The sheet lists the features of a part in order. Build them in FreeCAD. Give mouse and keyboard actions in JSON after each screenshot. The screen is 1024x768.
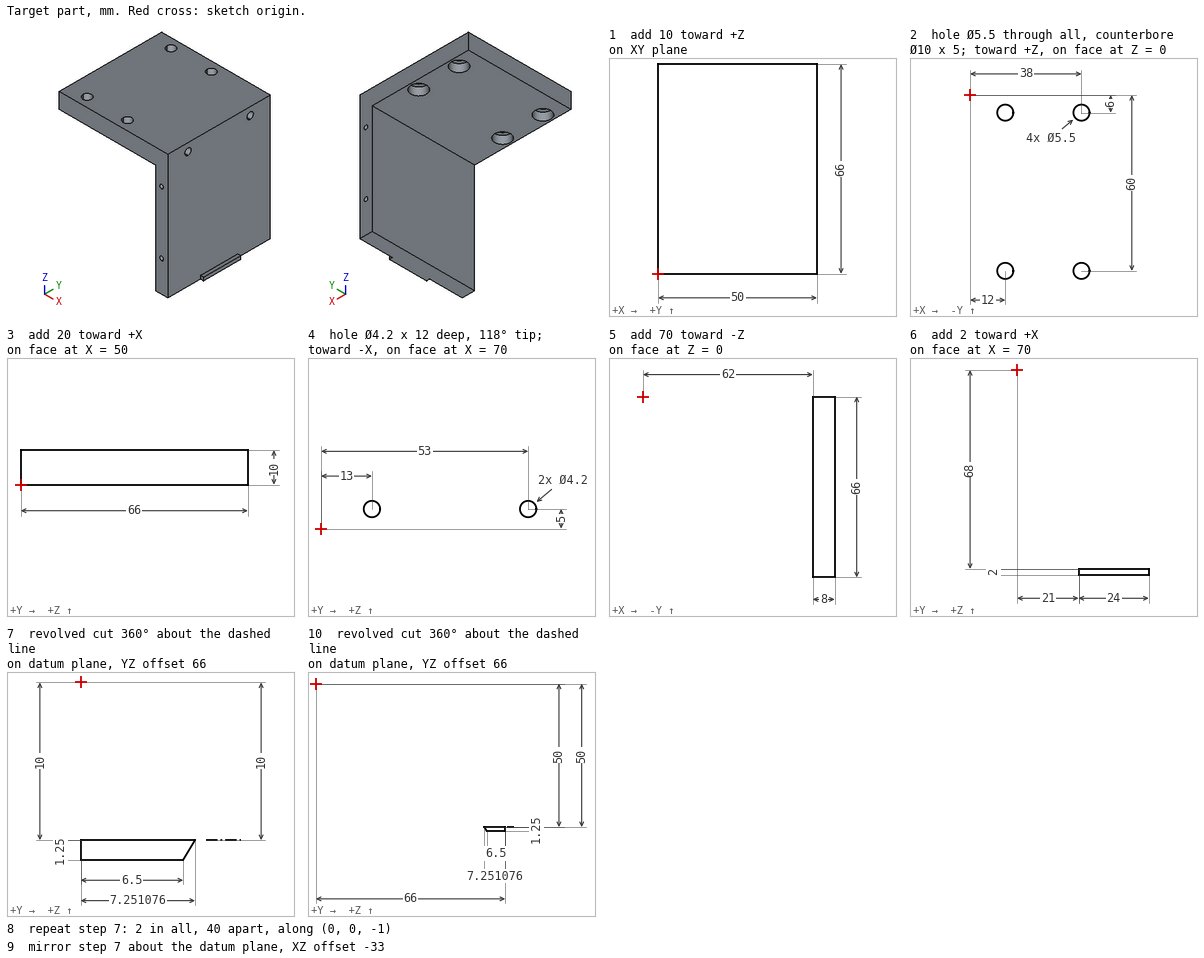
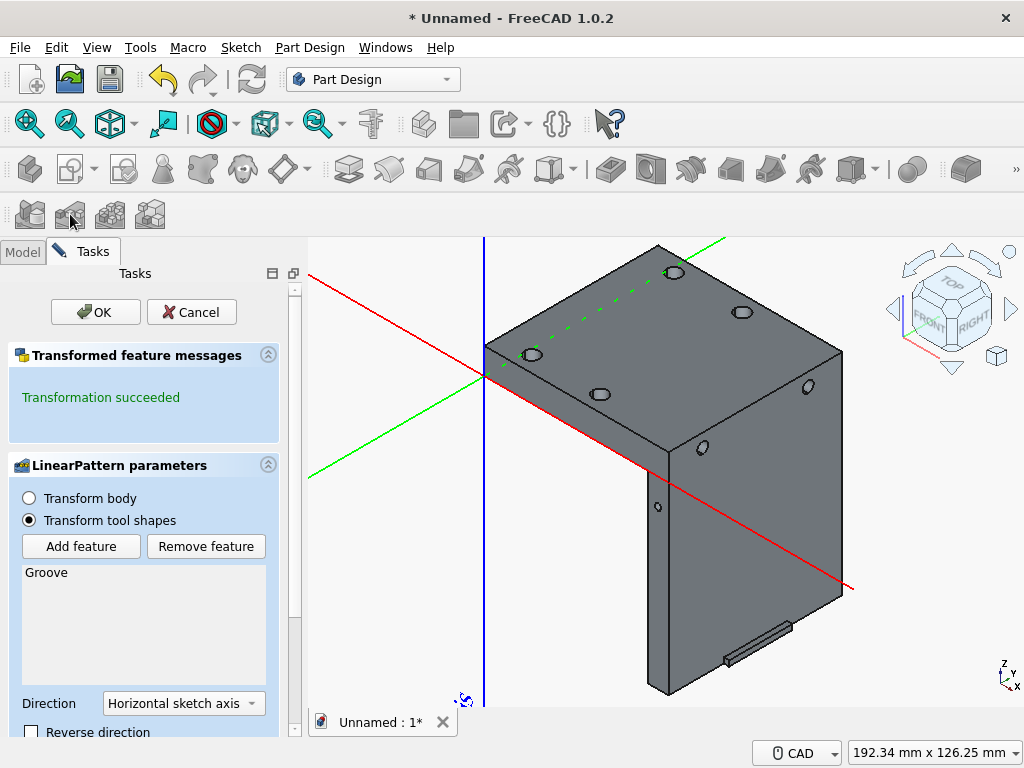
{"action": "left_click", "coordinate": [184, 704]}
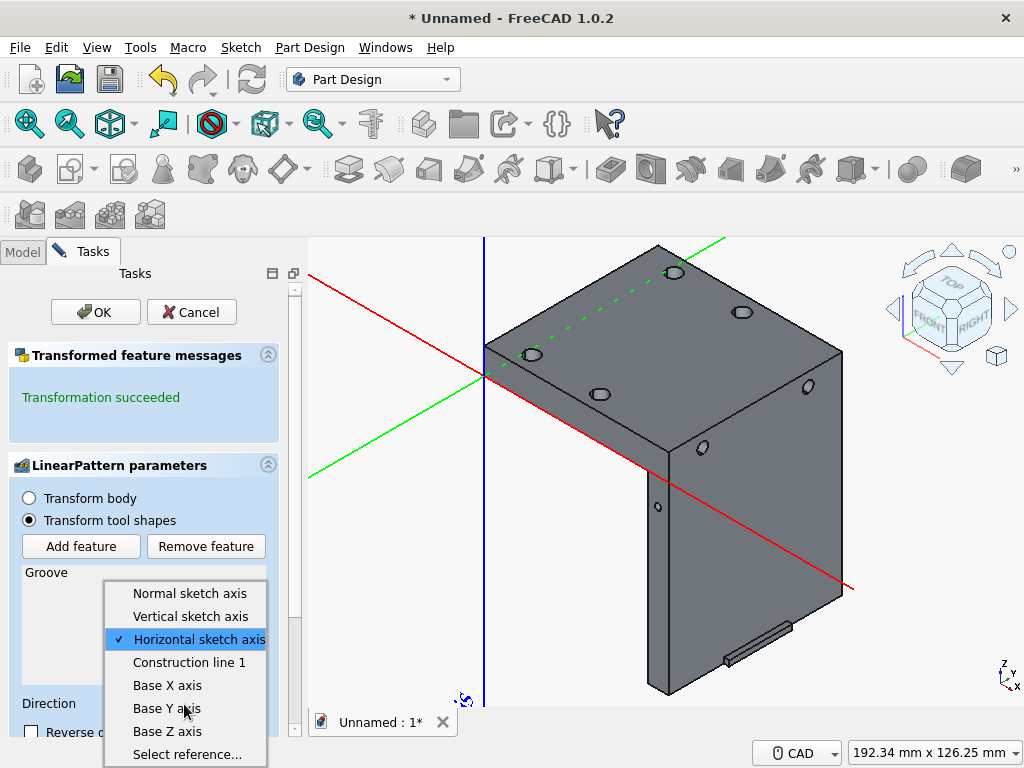
{"action": "left_click", "coordinate": [184, 732]}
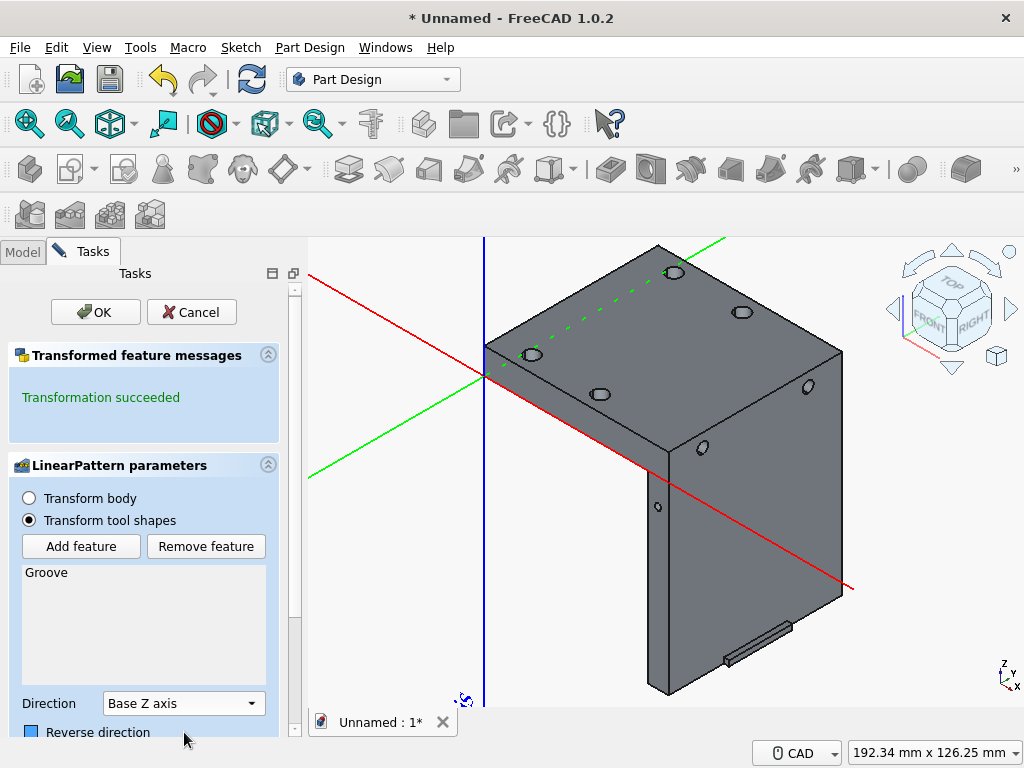
{"action": "scroll", "coordinate": [295, 510], "scroll_direction": "down", "scroll_amount": 2}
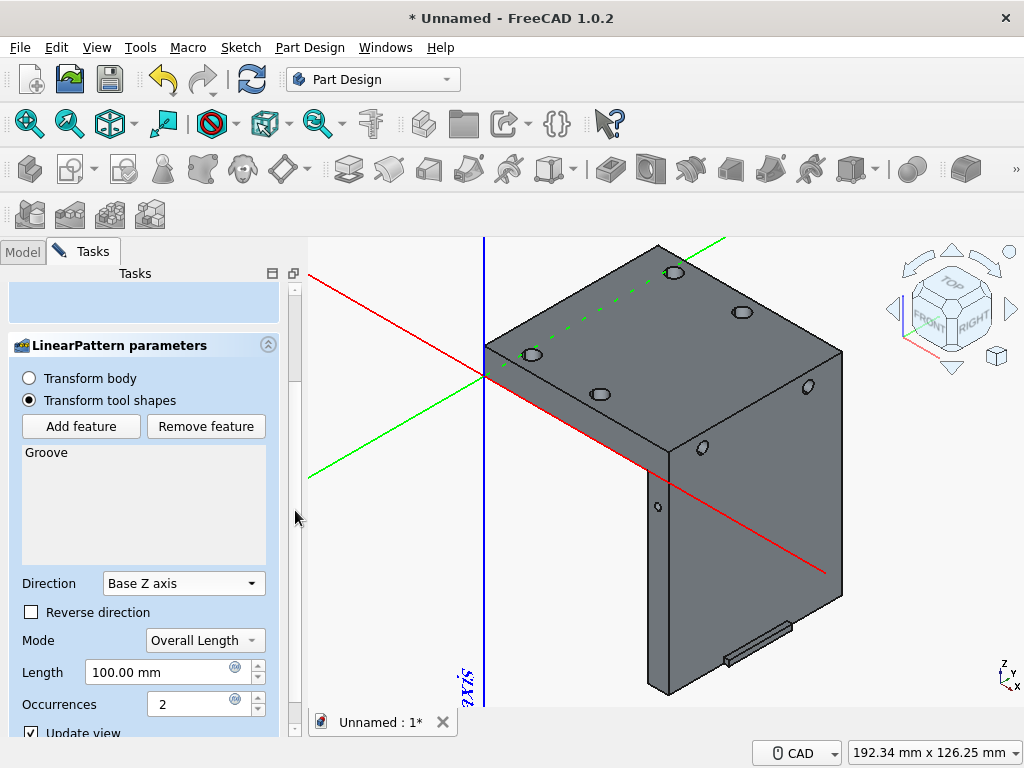
{"action": "left_click", "coordinate": [206, 640]}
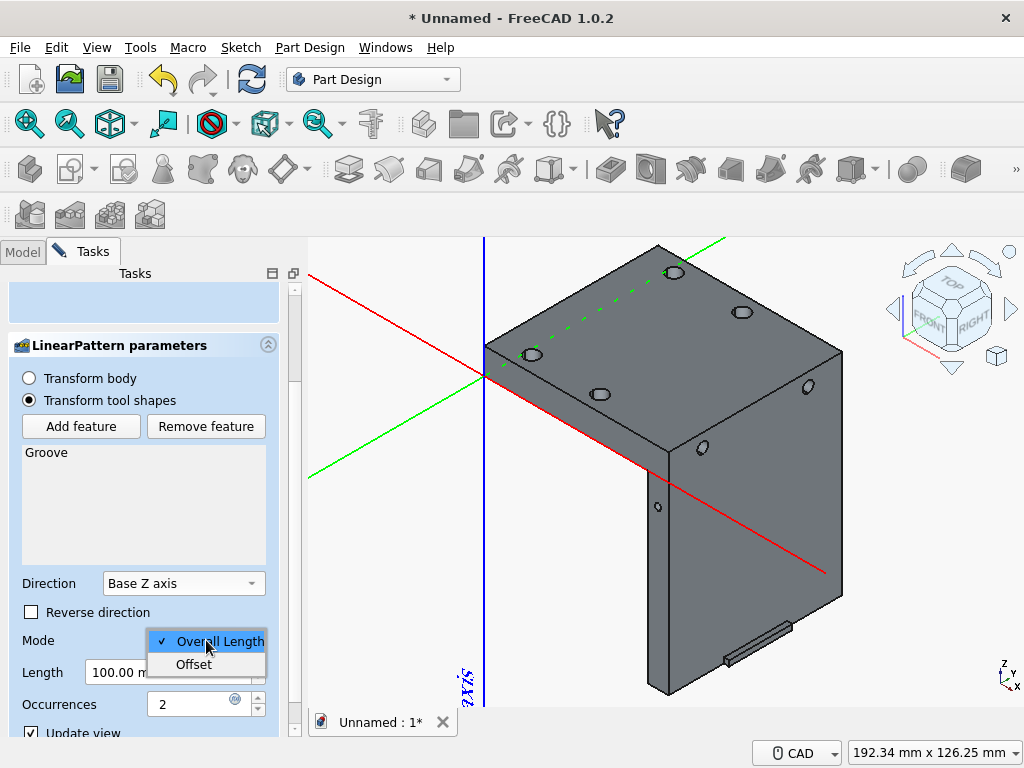
{"action": "left_click", "coordinate": [206, 664]}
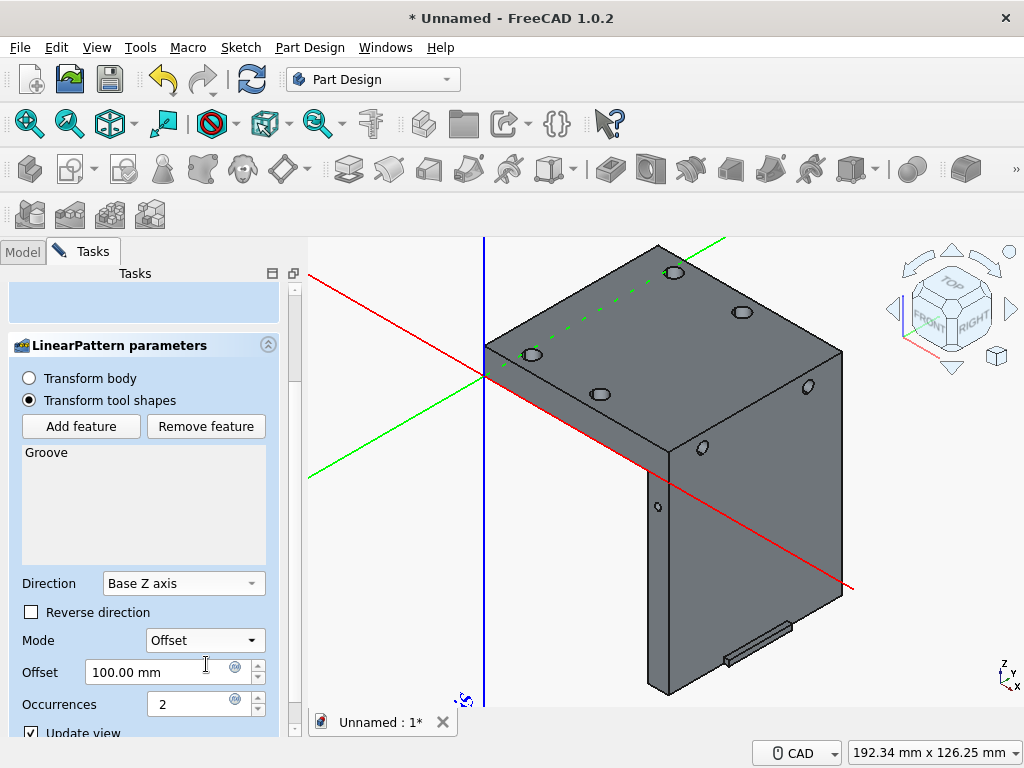
{"action": "triple_click", "coordinate": [168, 672]}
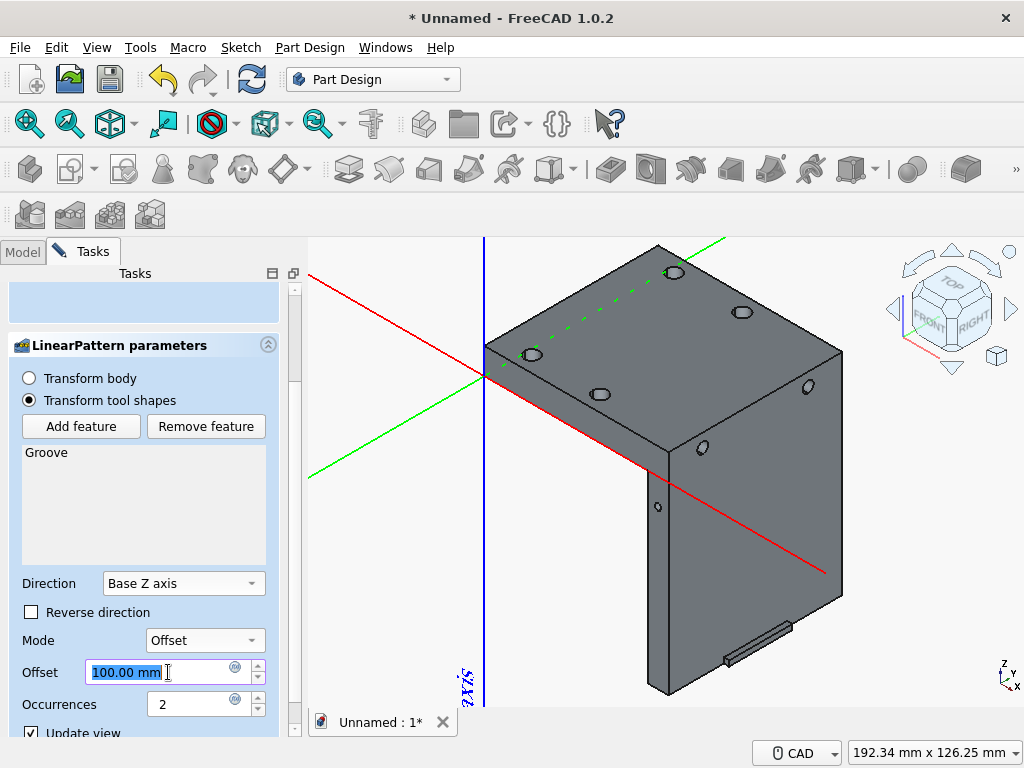
{"action": "type", "text": "40"}
{"action": "key", "text": "Tab"}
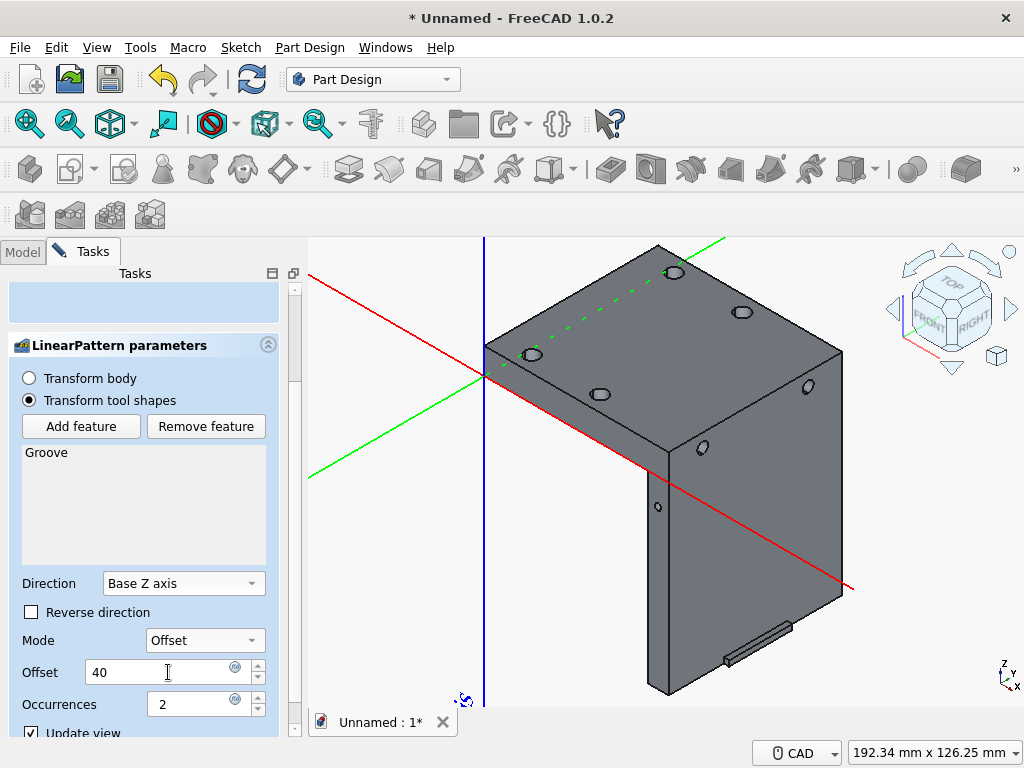
{"action": "triple_click", "coordinate": [198, 704]}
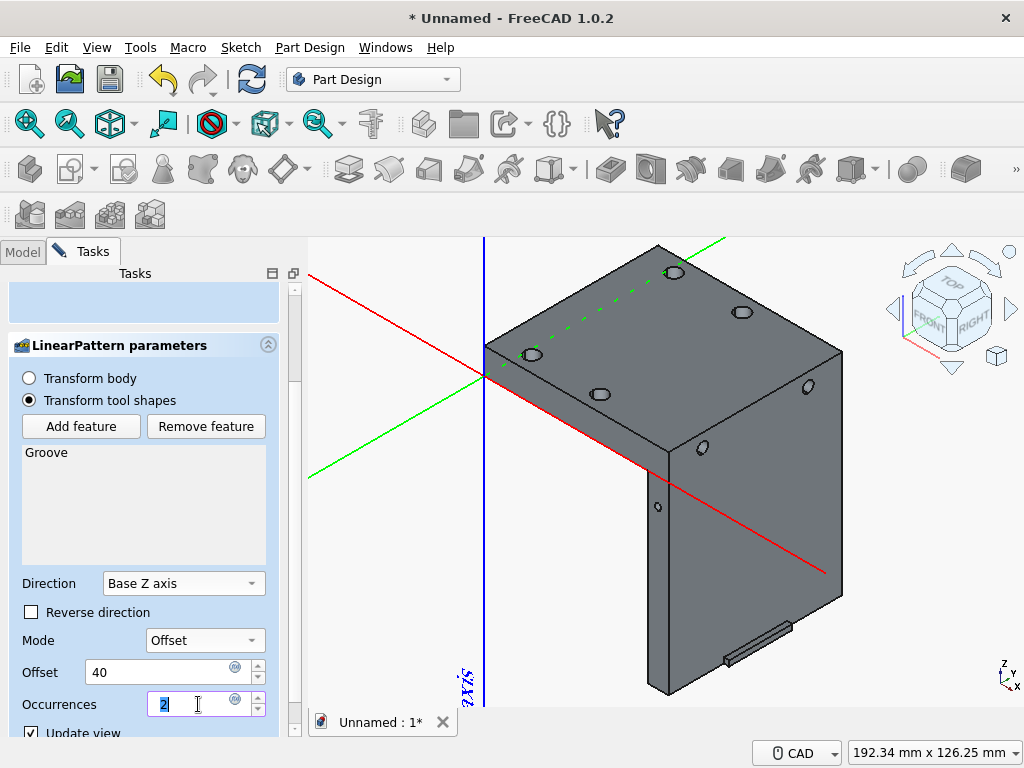
{"action": "type", "text": "2"}
{"action": "key", "text": "Tab"}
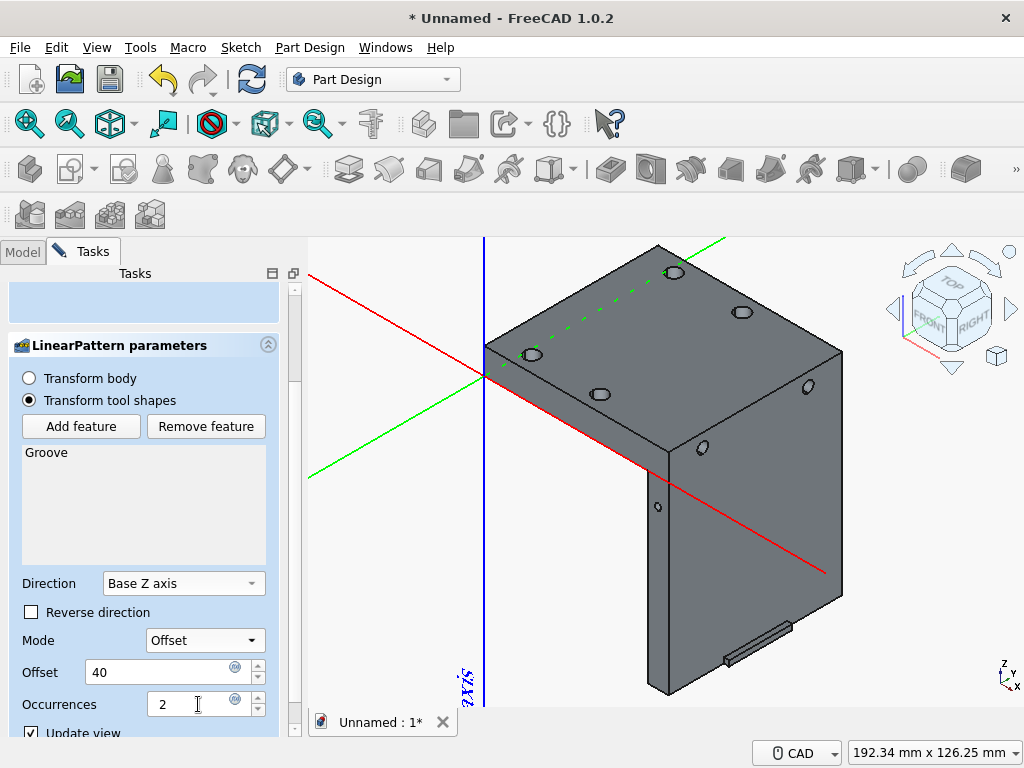
{"action": "left_click", "coordinate": [30, 612]}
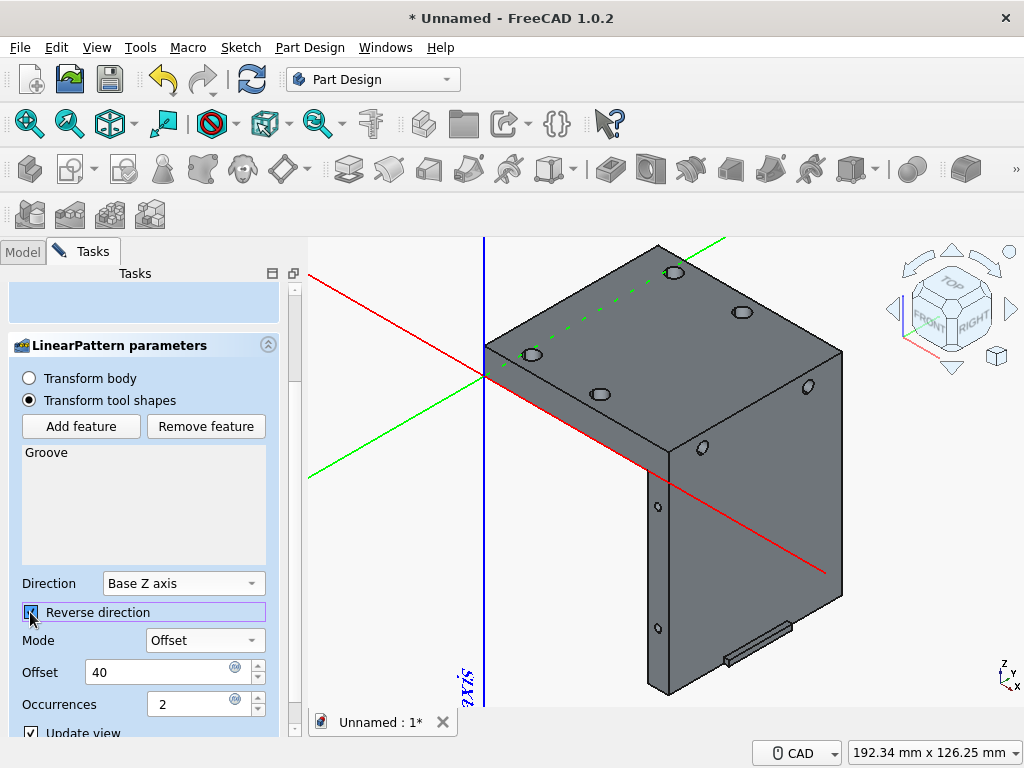
{"action": "scroll", "coordinate": [295, 510], "scroll_direction": "up", "scroll_amount": 3}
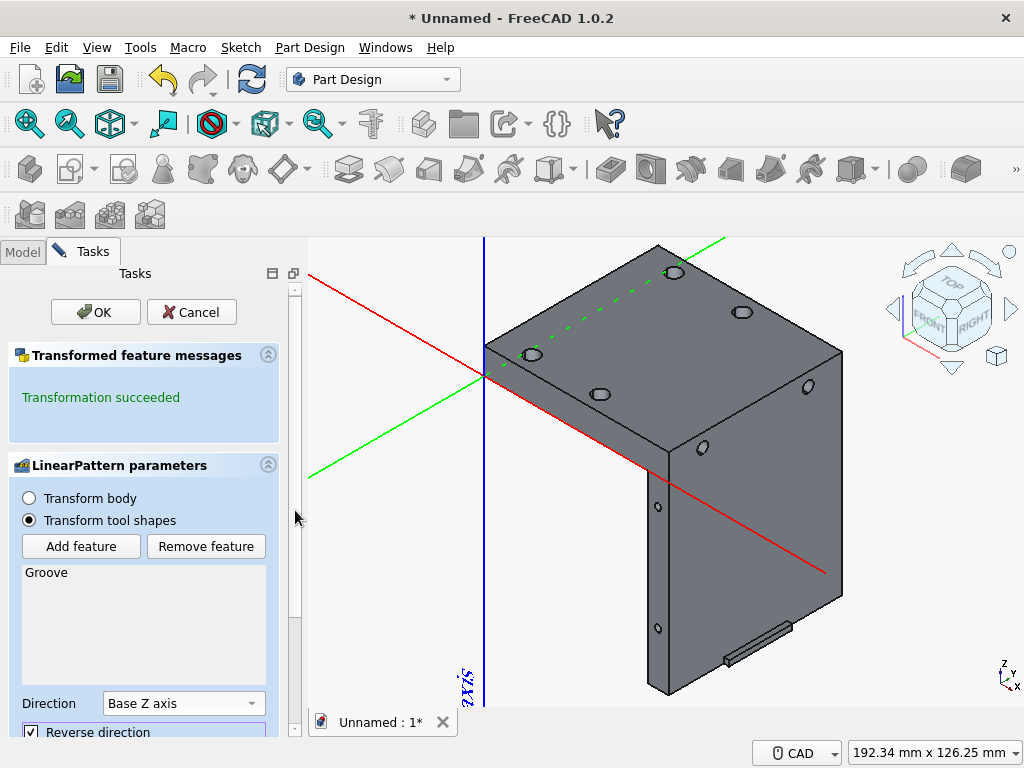
{"action": "left_click", "coordinate": [96, 312]}